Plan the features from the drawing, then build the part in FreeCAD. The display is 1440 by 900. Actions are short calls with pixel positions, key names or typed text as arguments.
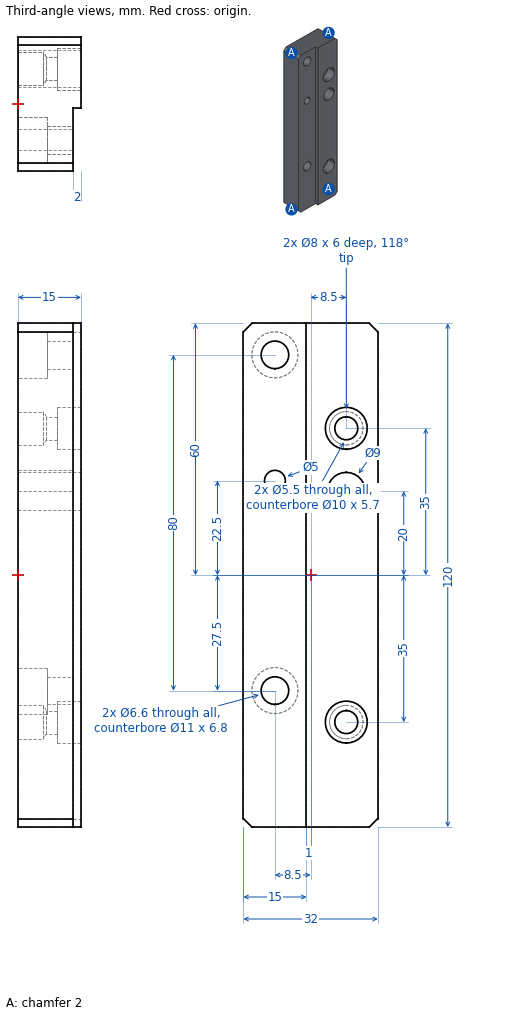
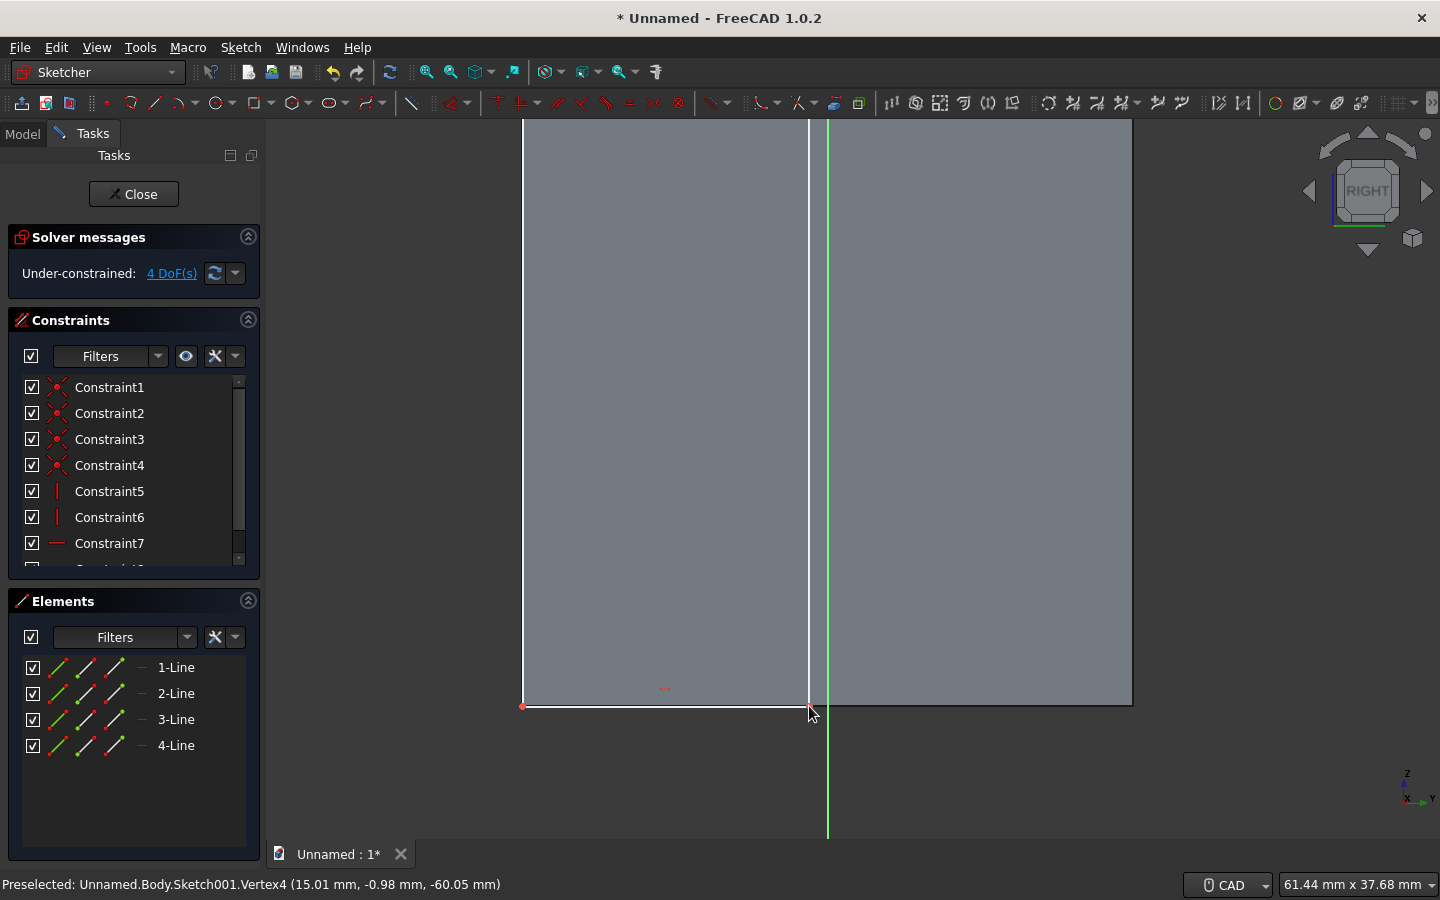
click(450, 104)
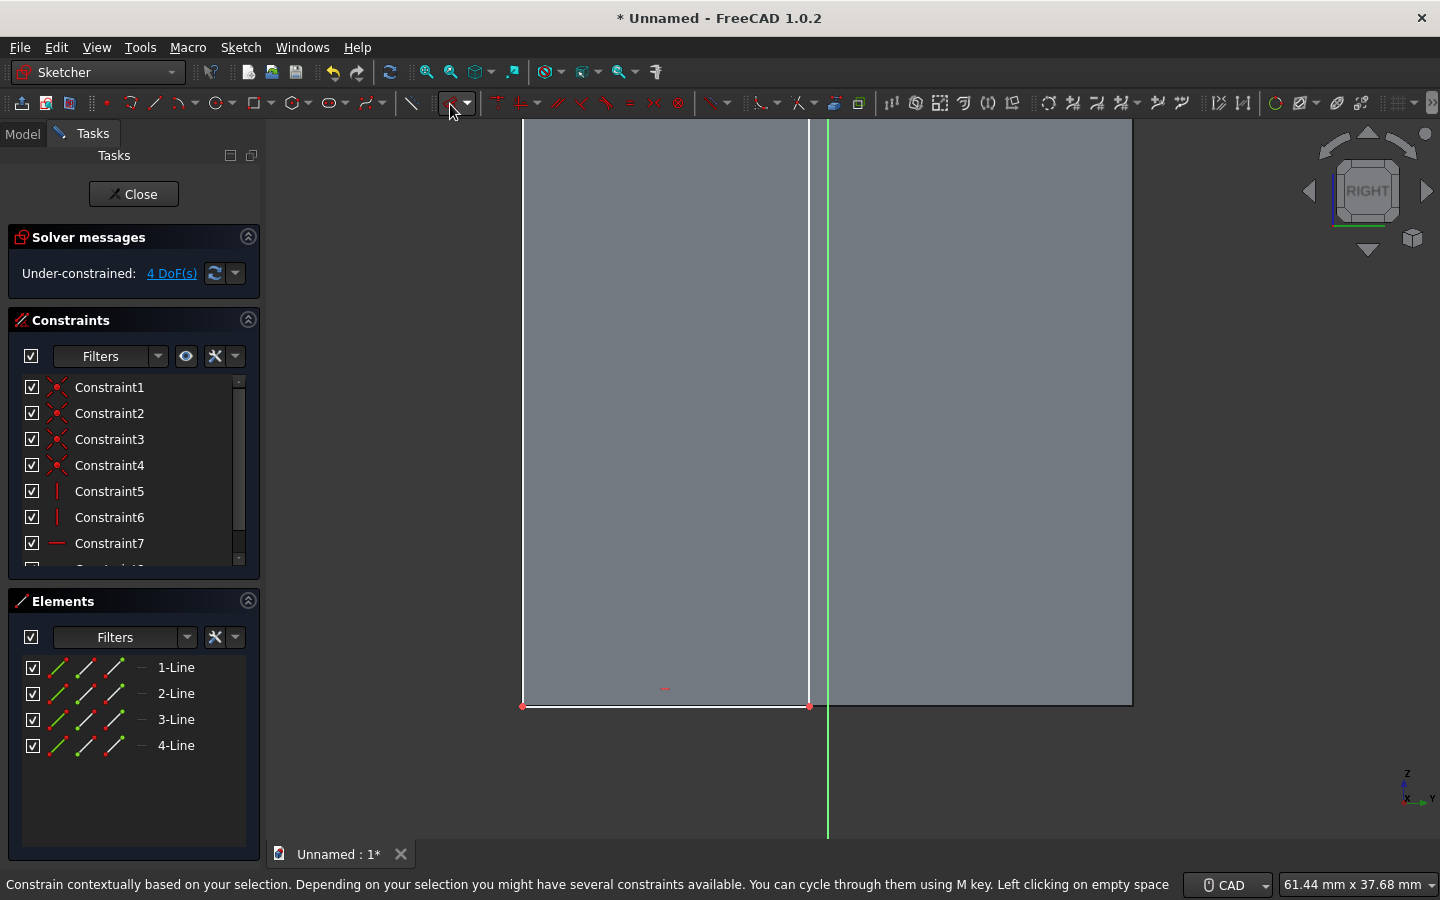
scroll(812, 712, down, 8)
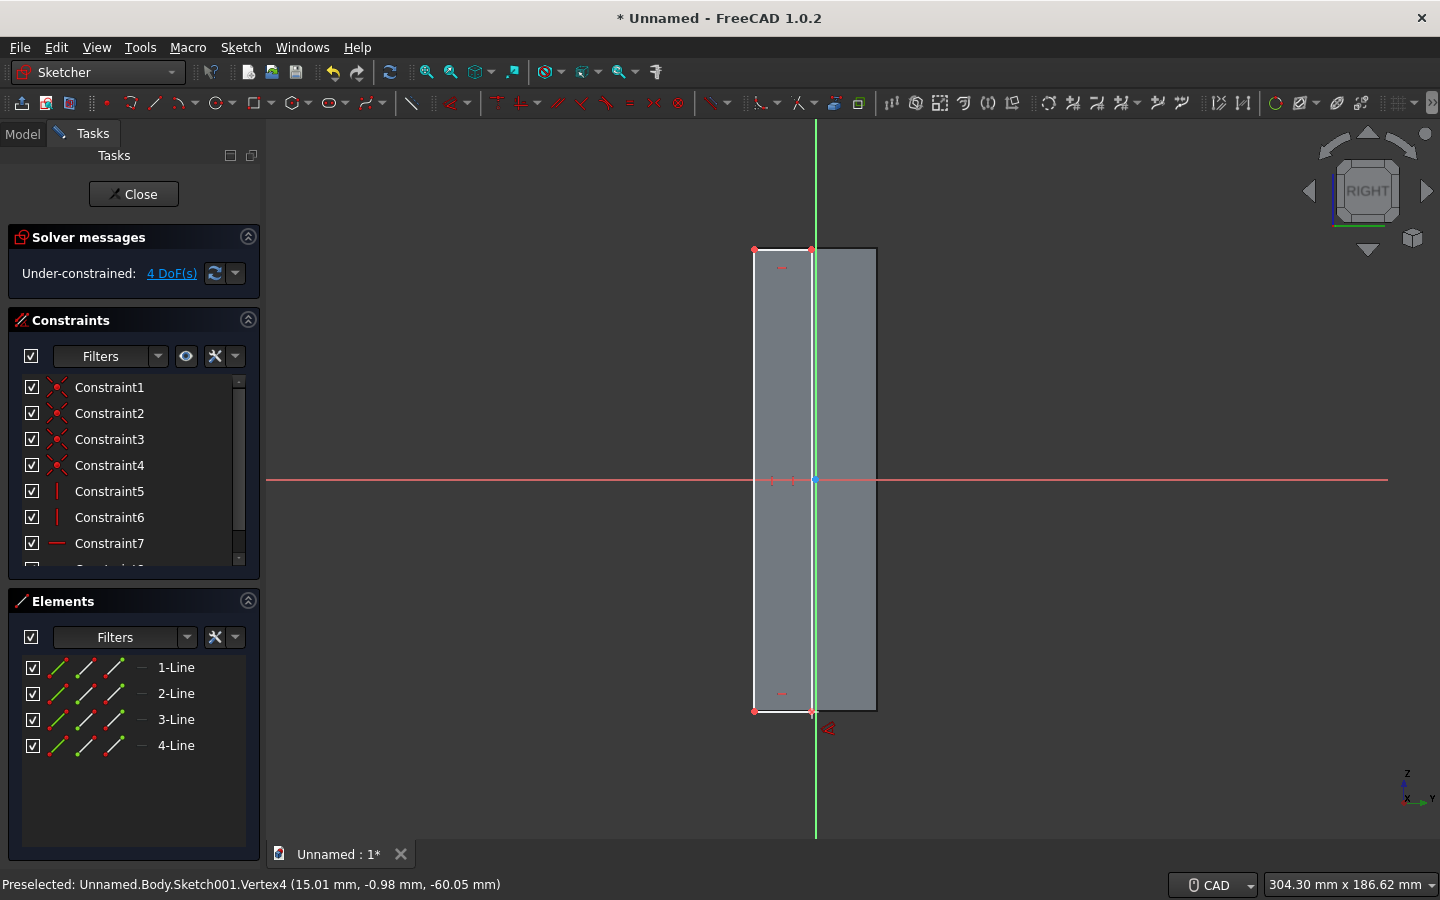
click(771, 712)
click(783, 746)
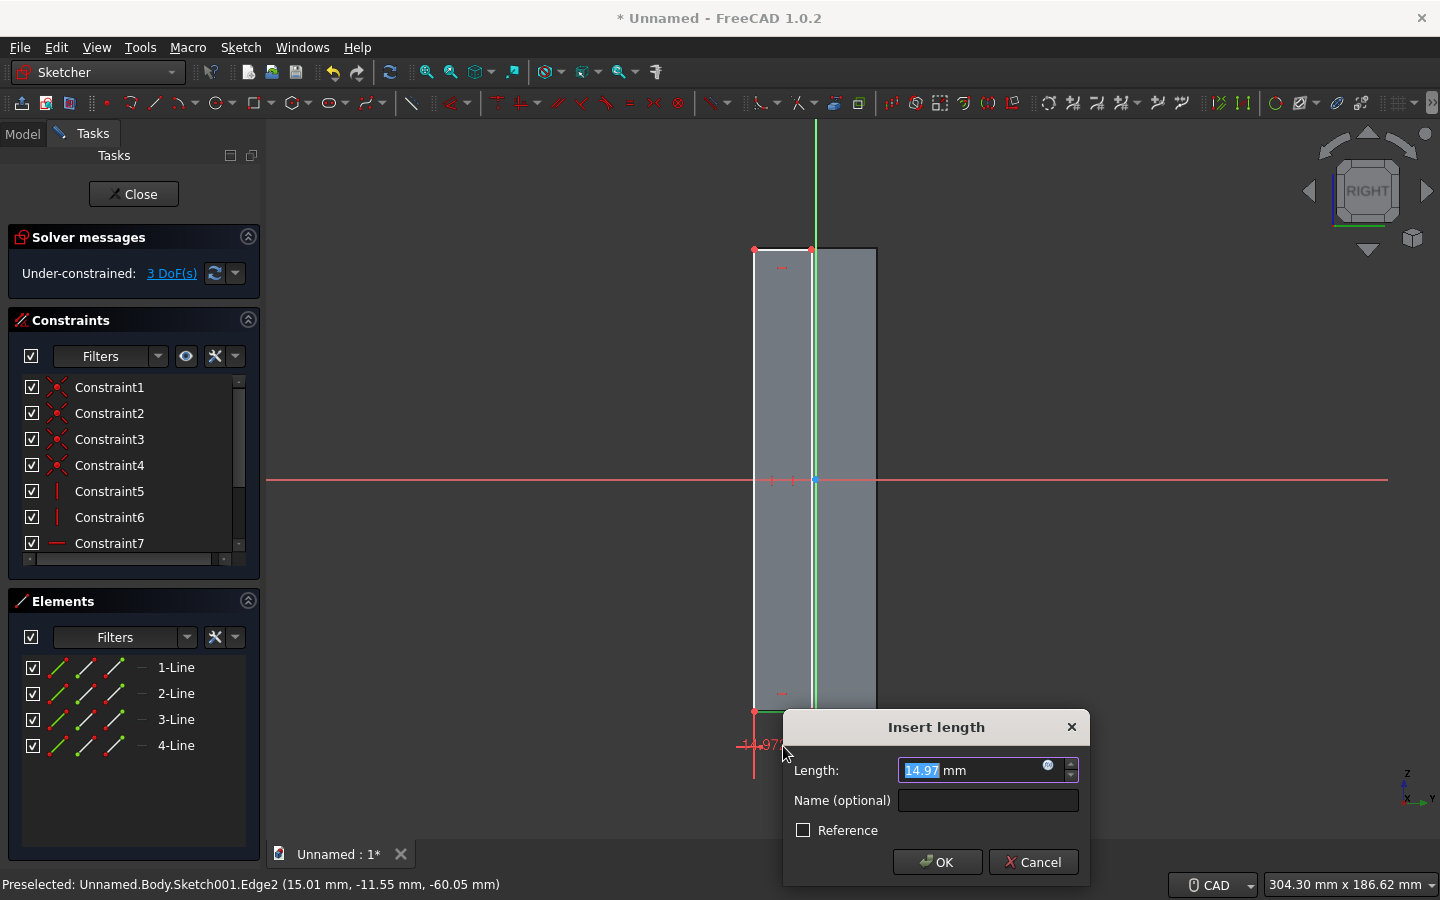
text(15)
key(Return)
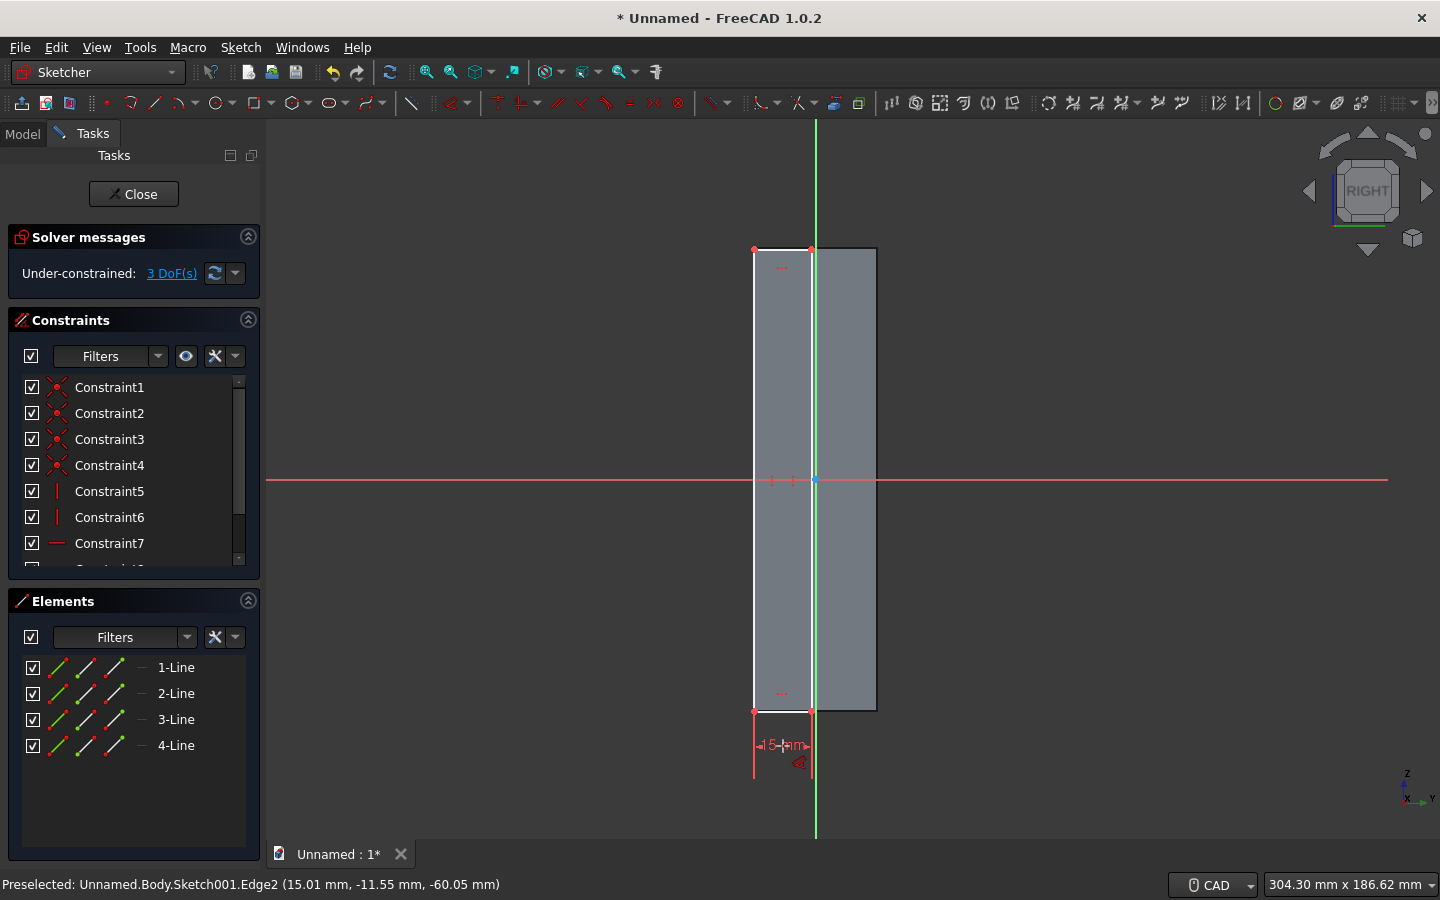
scroll(812, 712, up, 12)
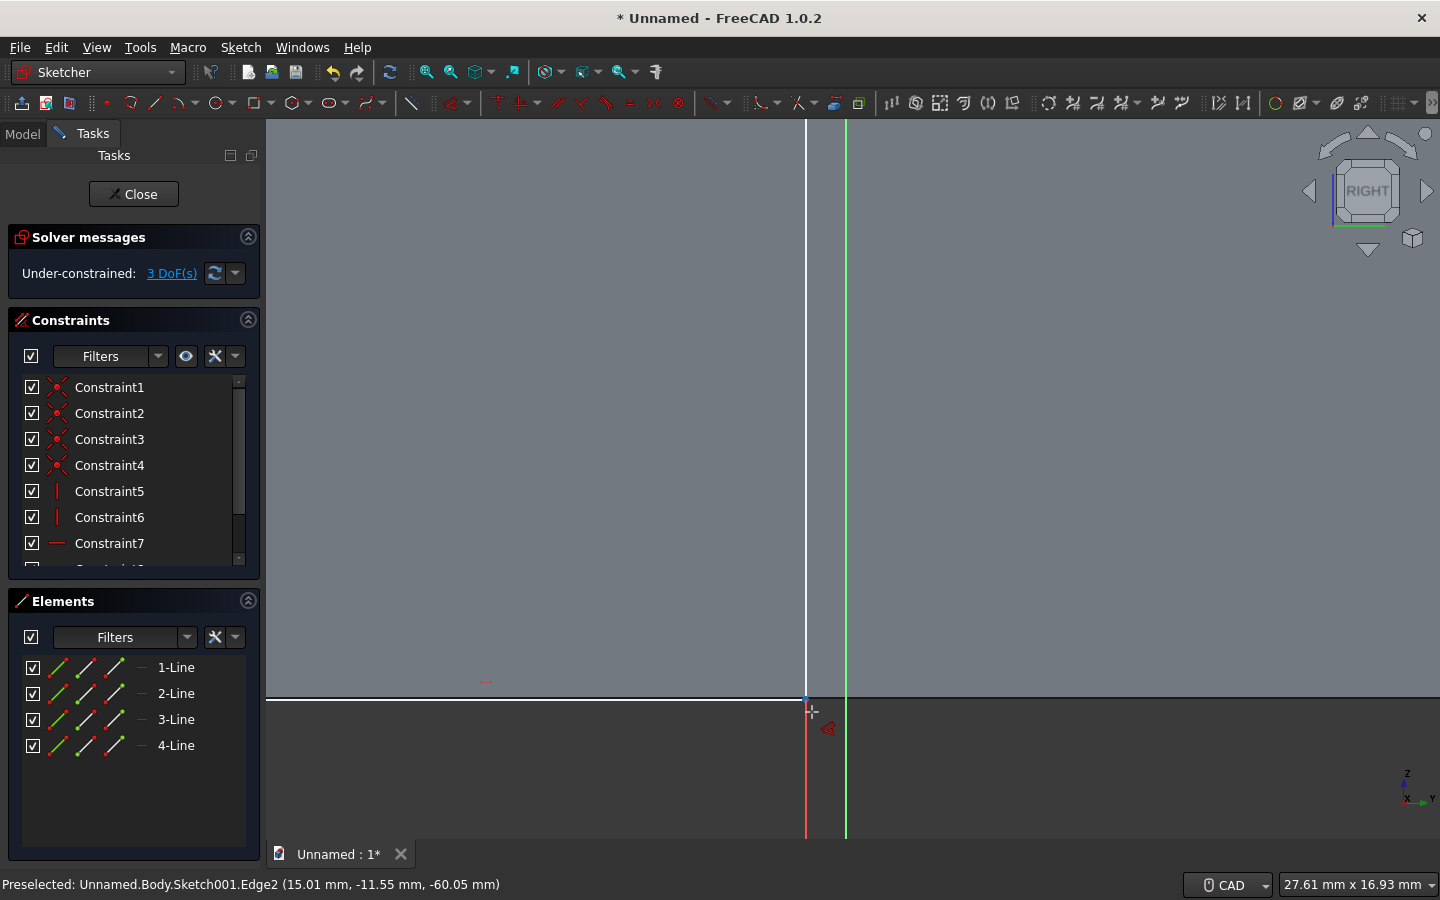
click(806, 700)
click(826, 734)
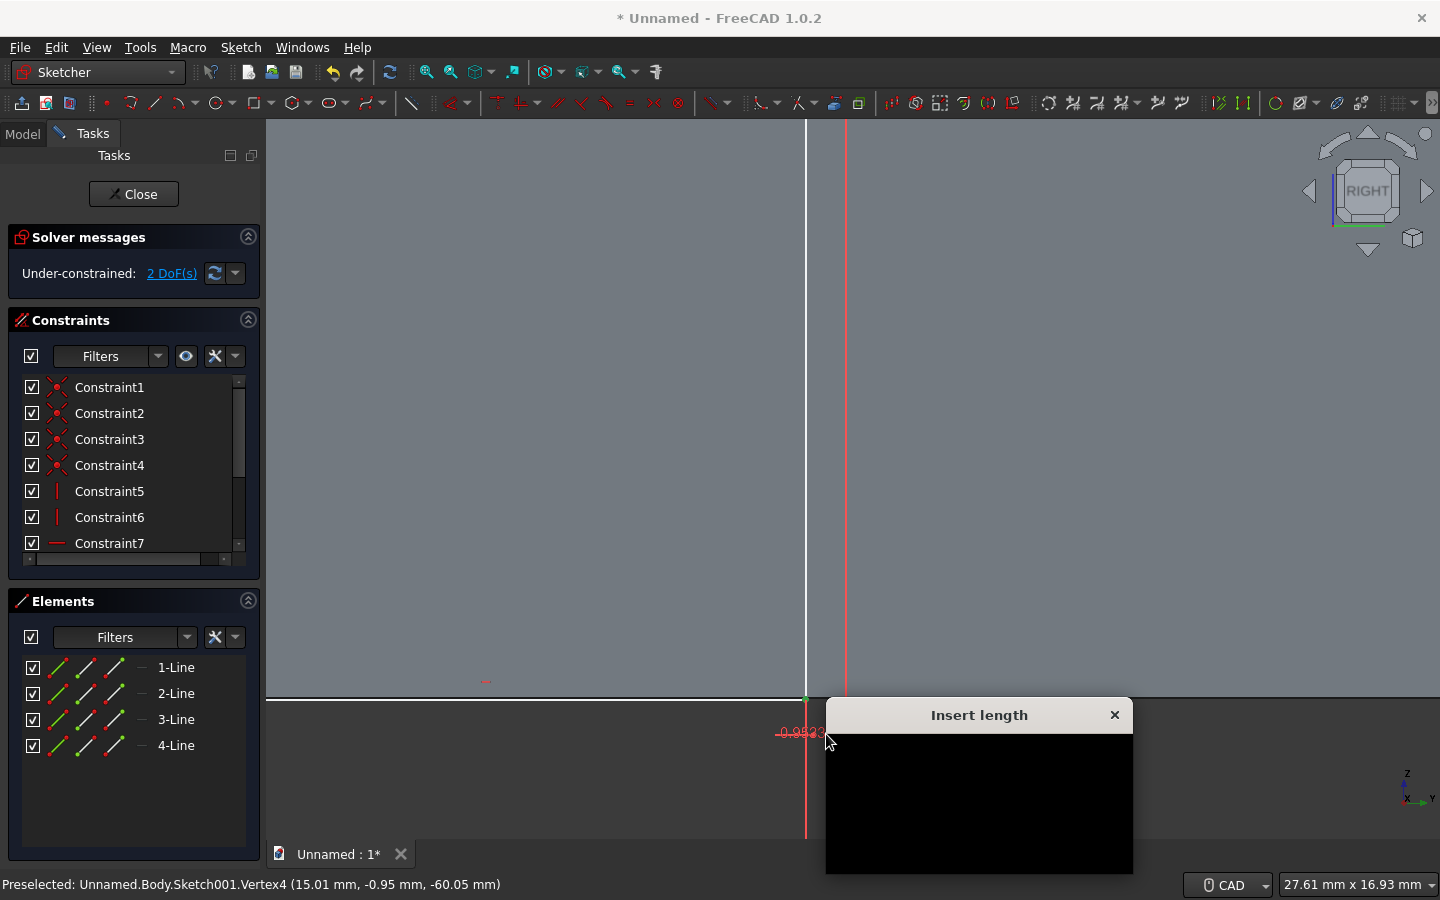
text(1)
key(Return)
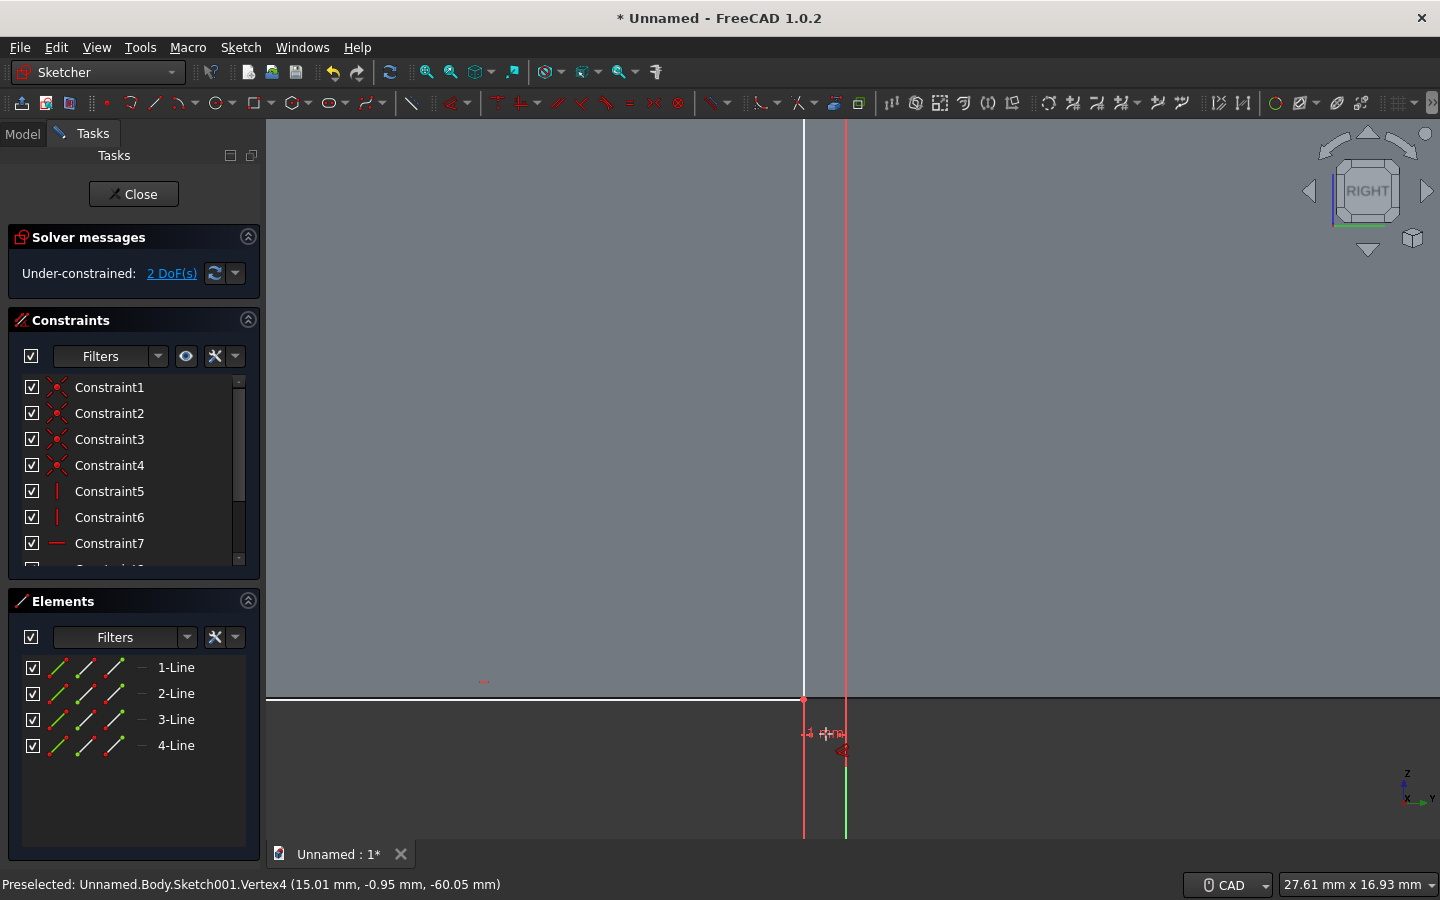
scroll(812, 712, down, 12)